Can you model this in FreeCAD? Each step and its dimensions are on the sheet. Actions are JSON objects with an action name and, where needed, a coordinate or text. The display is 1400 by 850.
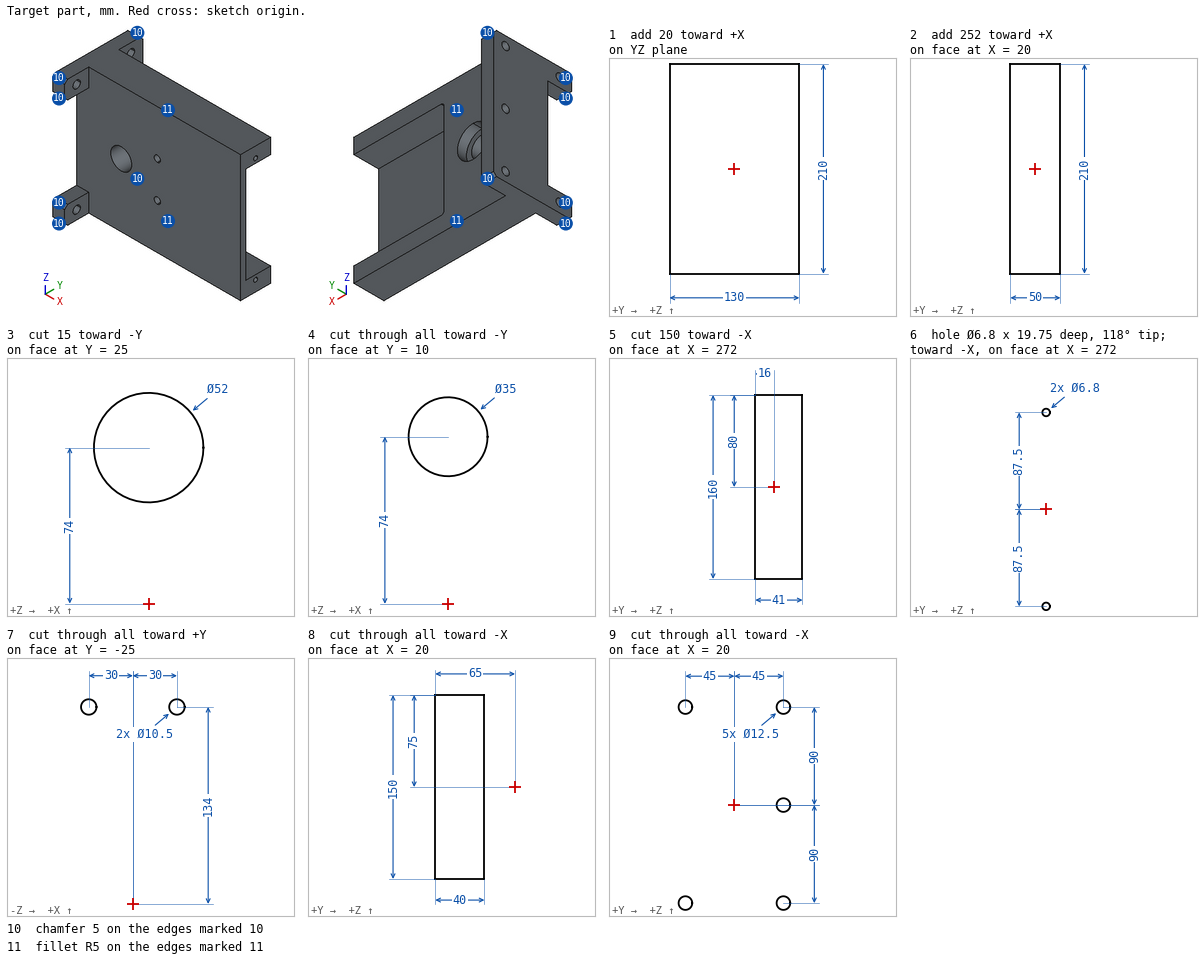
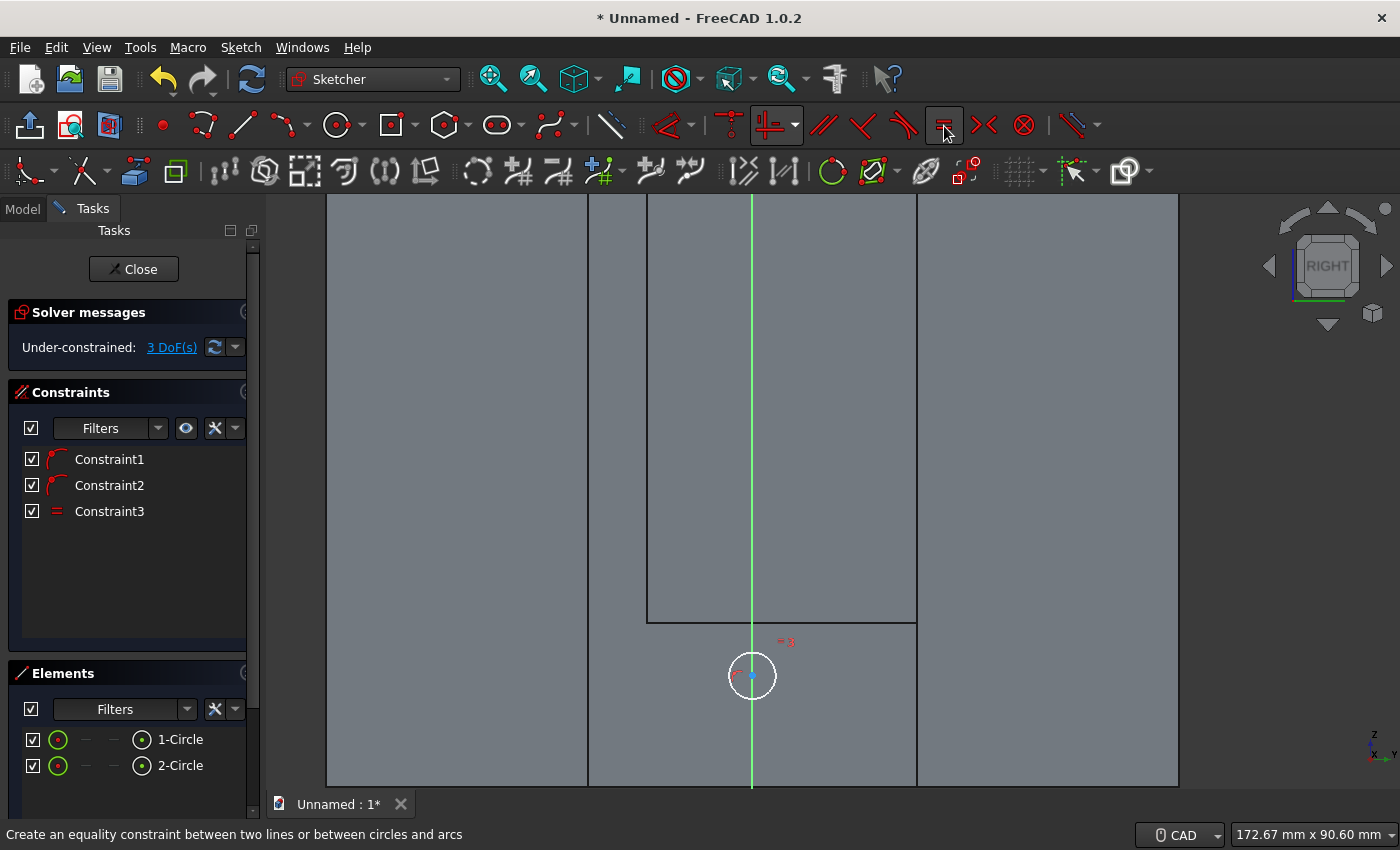
{"action": "left_click", "coordinate": [666, 126]}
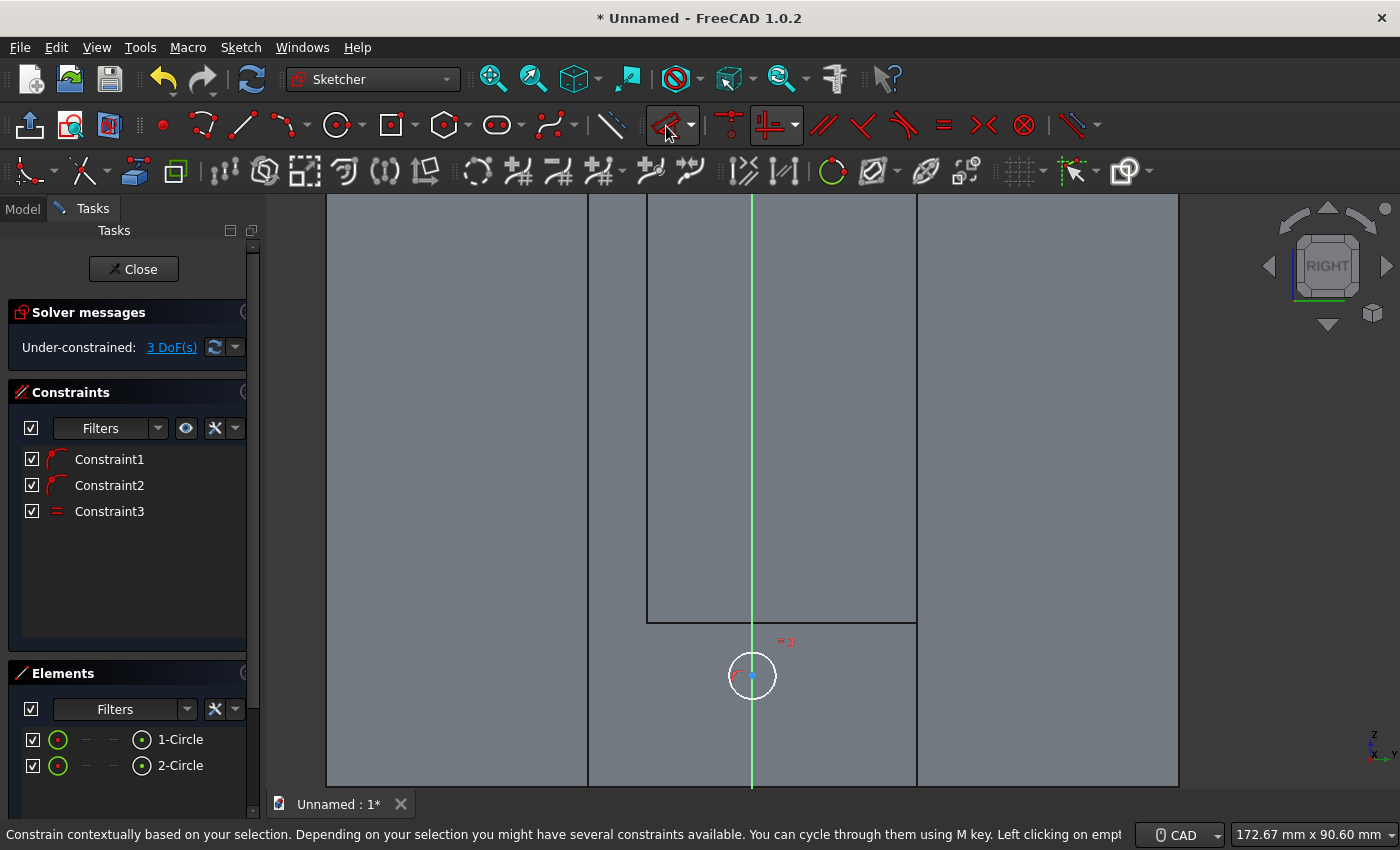
{"action": "scroll", "coordinate": [770, 661], "scroll_direction": "down", "scroll_amount": 6}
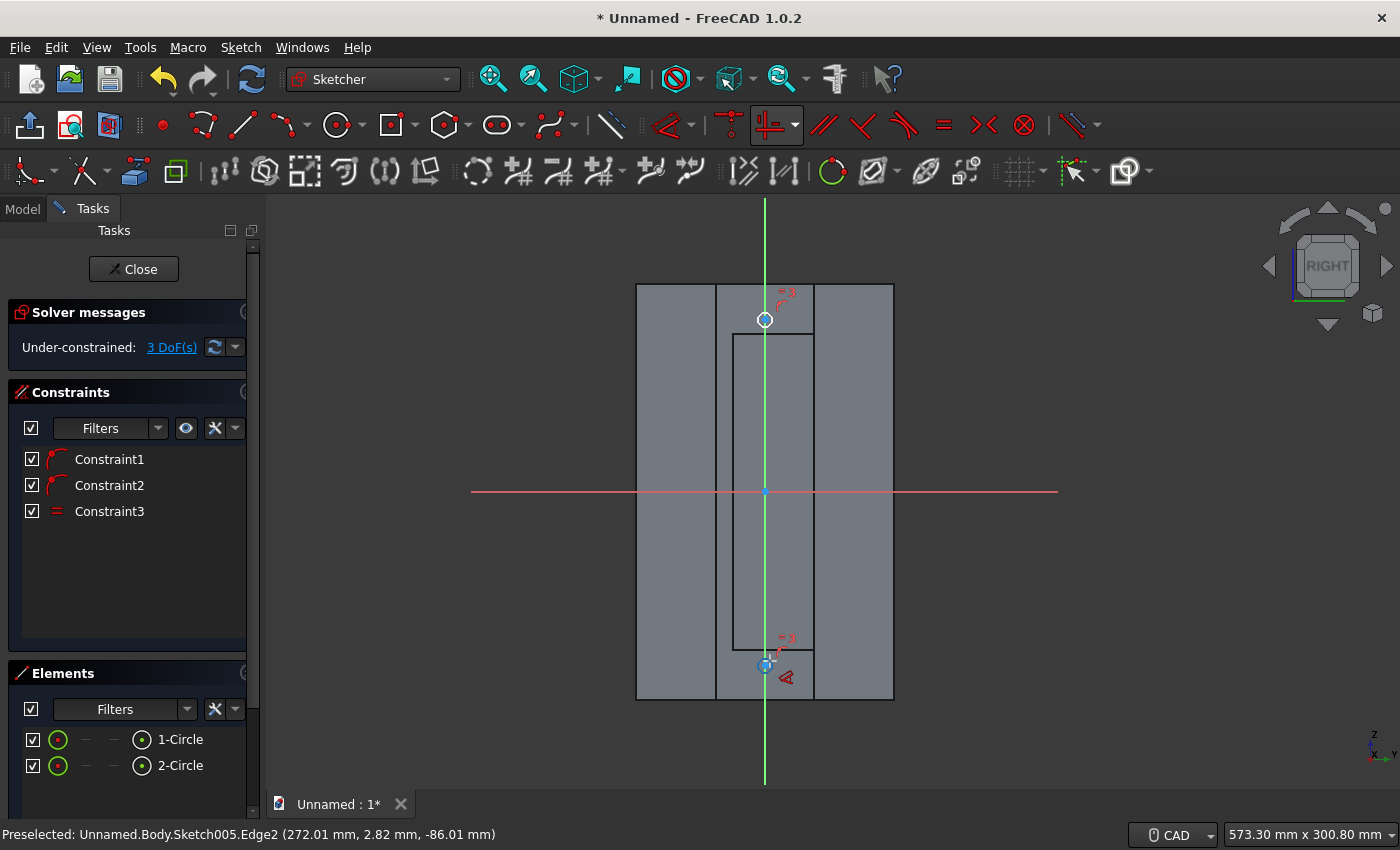
{"action": "scroll", "coordinate": [770, 315], "scroll_direction": "up", "scroll_amount": 6}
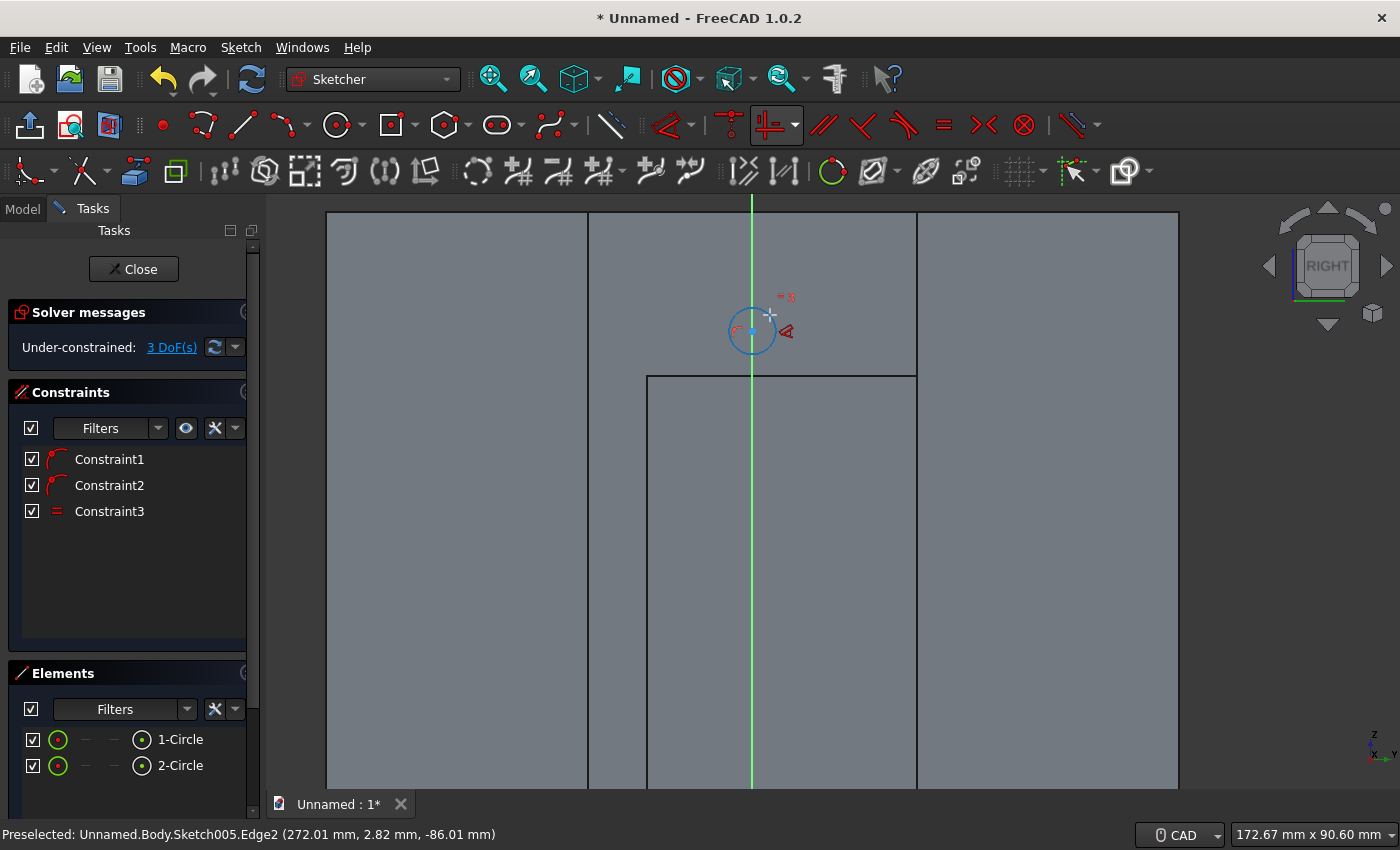
{"action": "left_click", "coordinate": [769, 315]}
{"action": "left_click", "coordinate": [792, 293]}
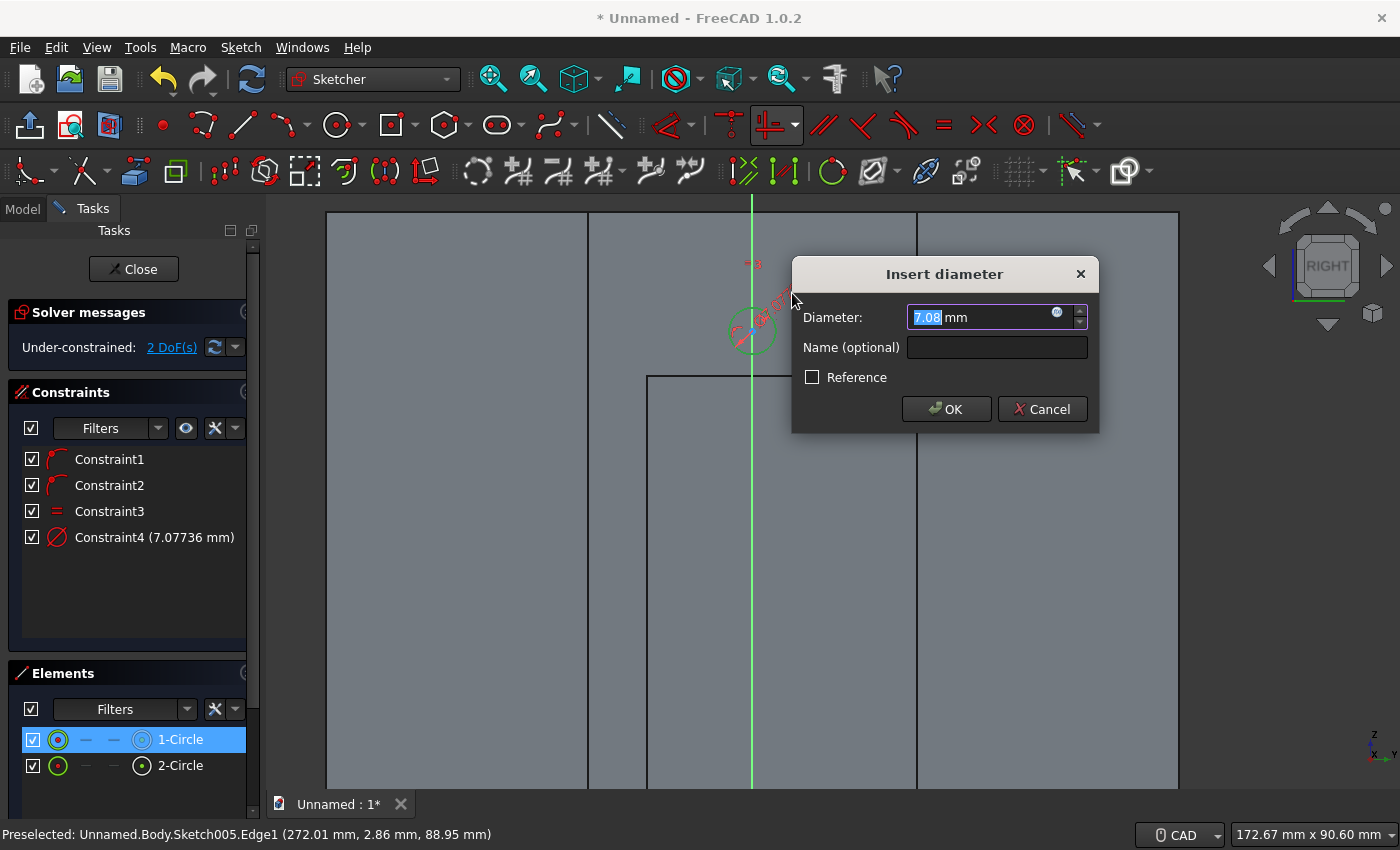
{"action": "type", "text": "6.8"}
{"action": "key", "text": "Return"}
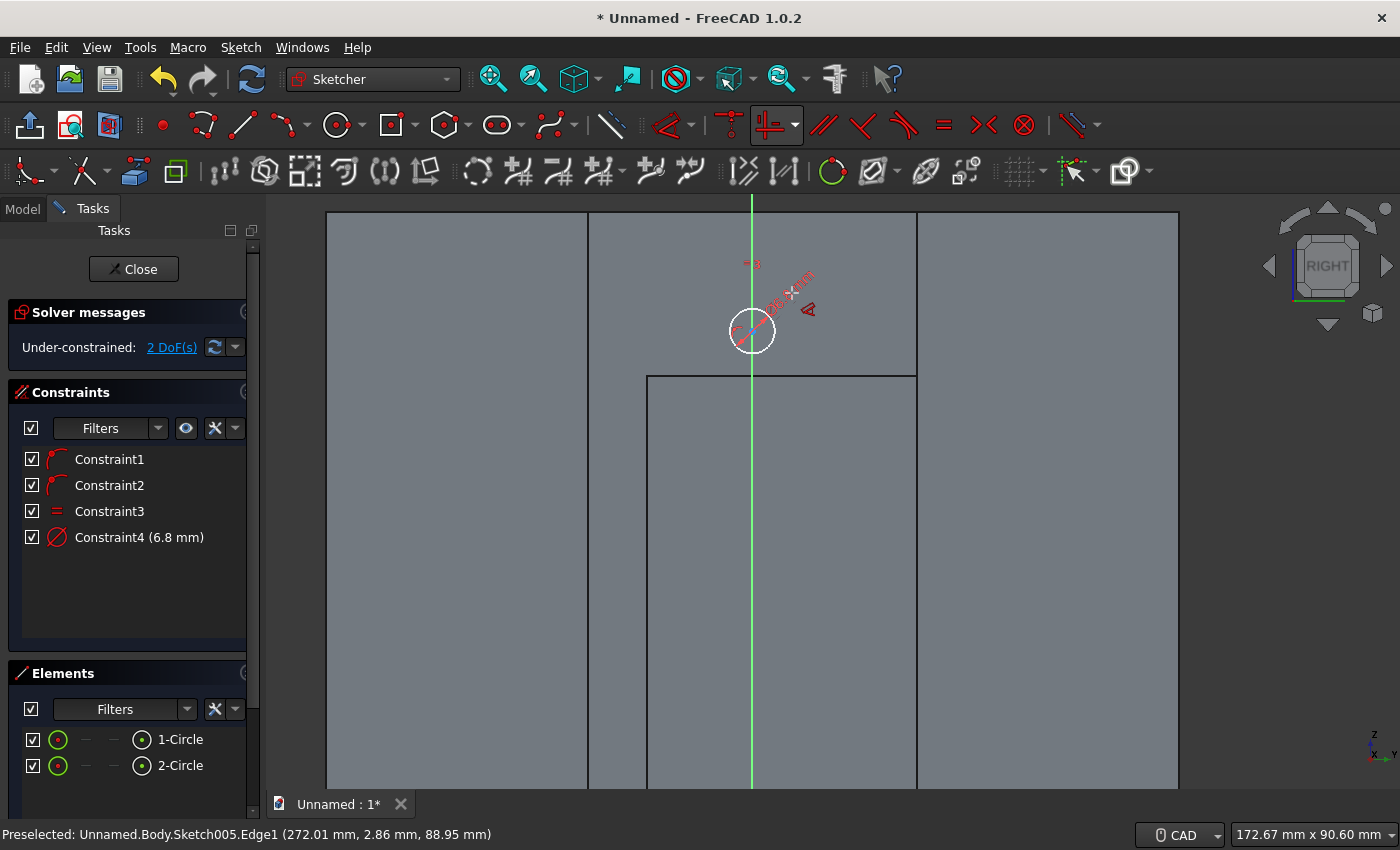
{"action": "scroll", "coordinate": [770, 315], "scroll_direction": "down", "scroll_amount": 6}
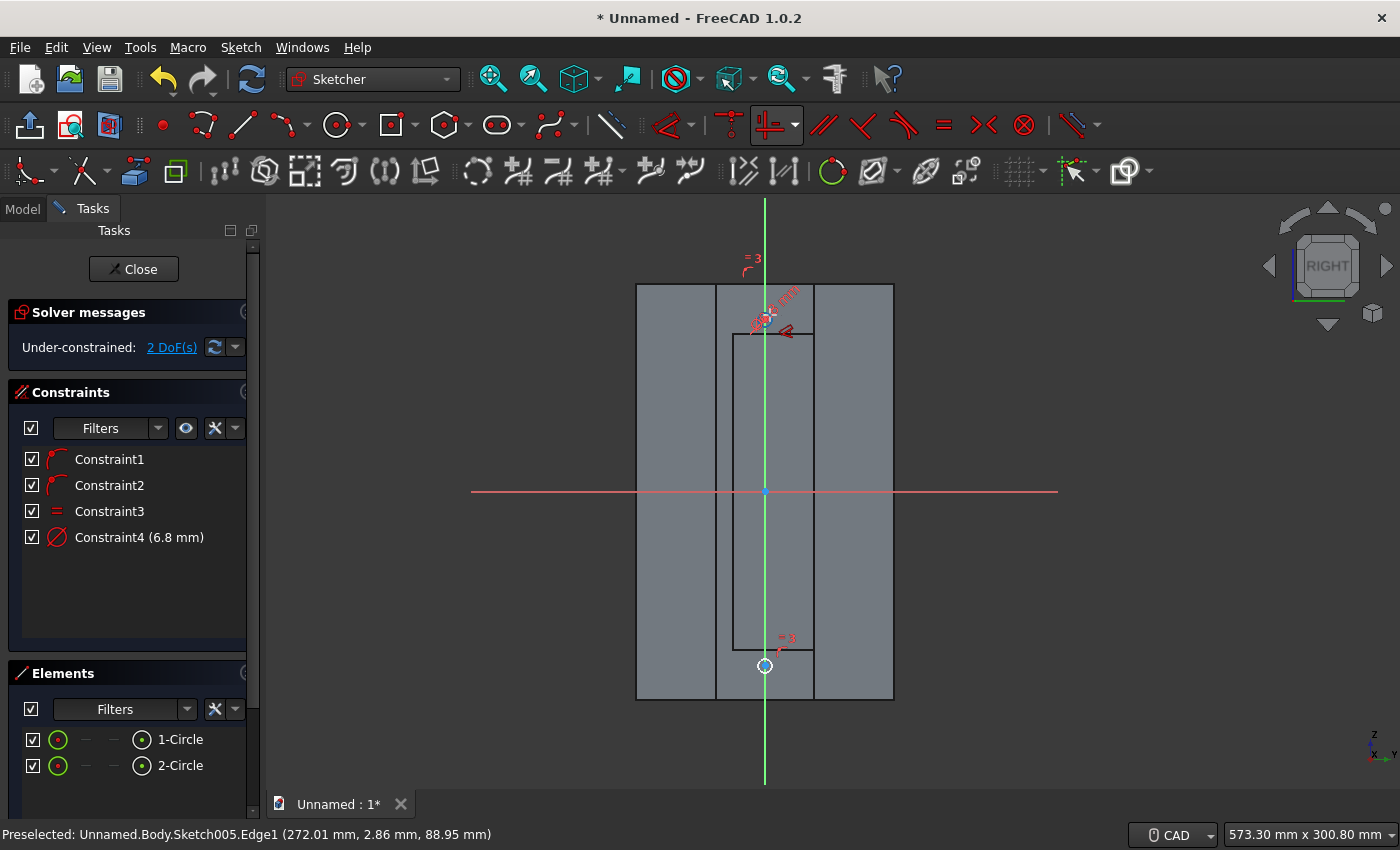
{"action": "left_click", "coordinate": [765, 320]}
{"action": "left_click", "coordinate": [799, 406]}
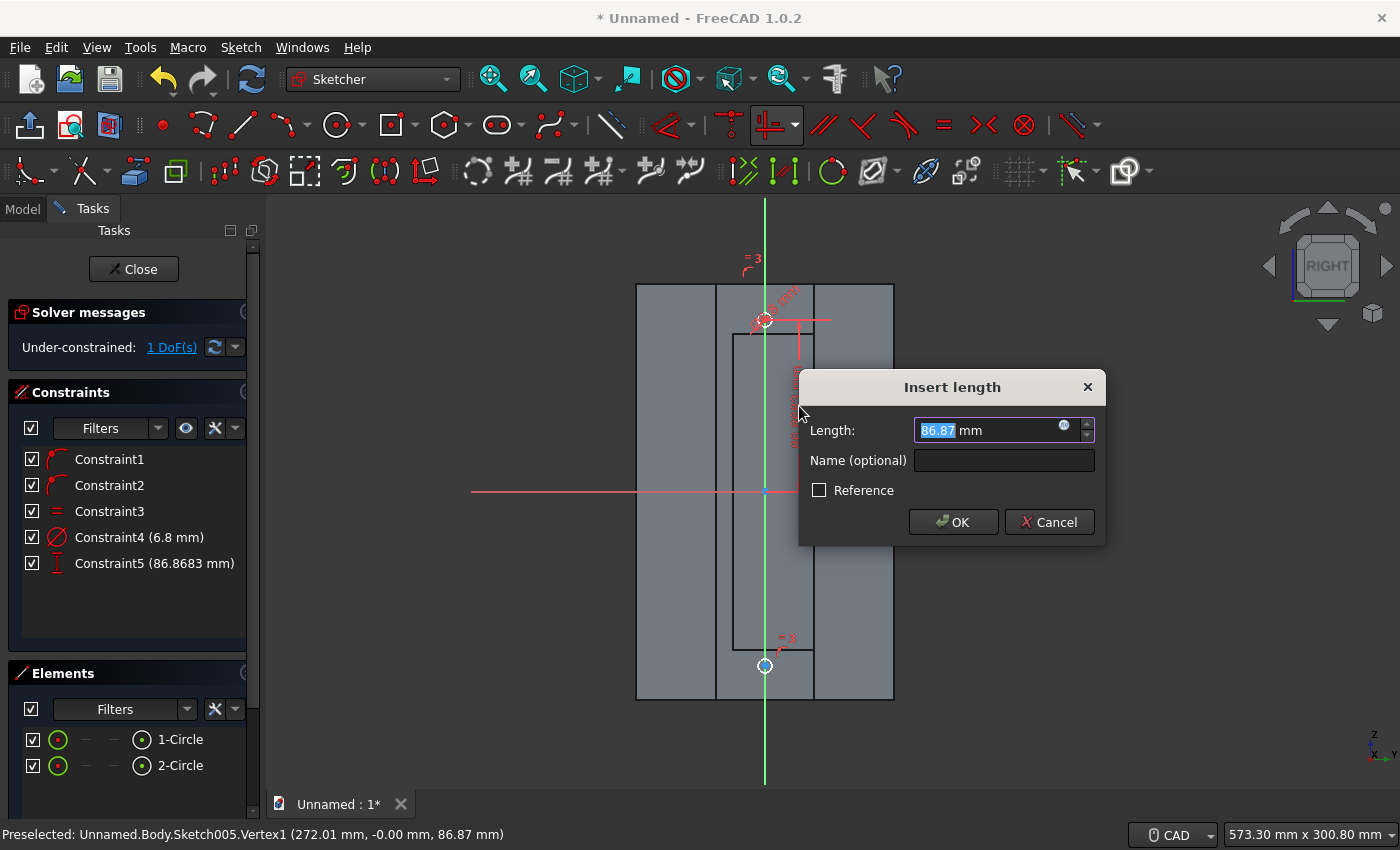
{"action": "type", "text": "87.5"}
{"action": "key", "text": "Return"}